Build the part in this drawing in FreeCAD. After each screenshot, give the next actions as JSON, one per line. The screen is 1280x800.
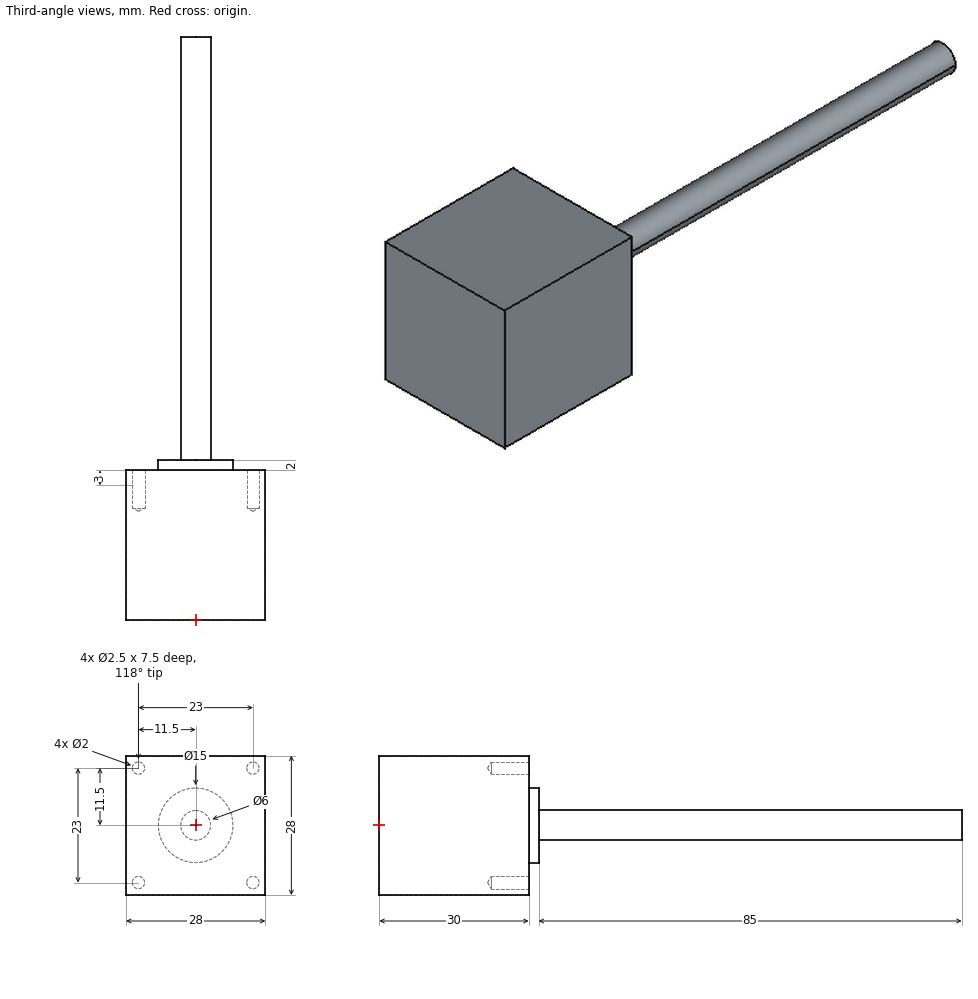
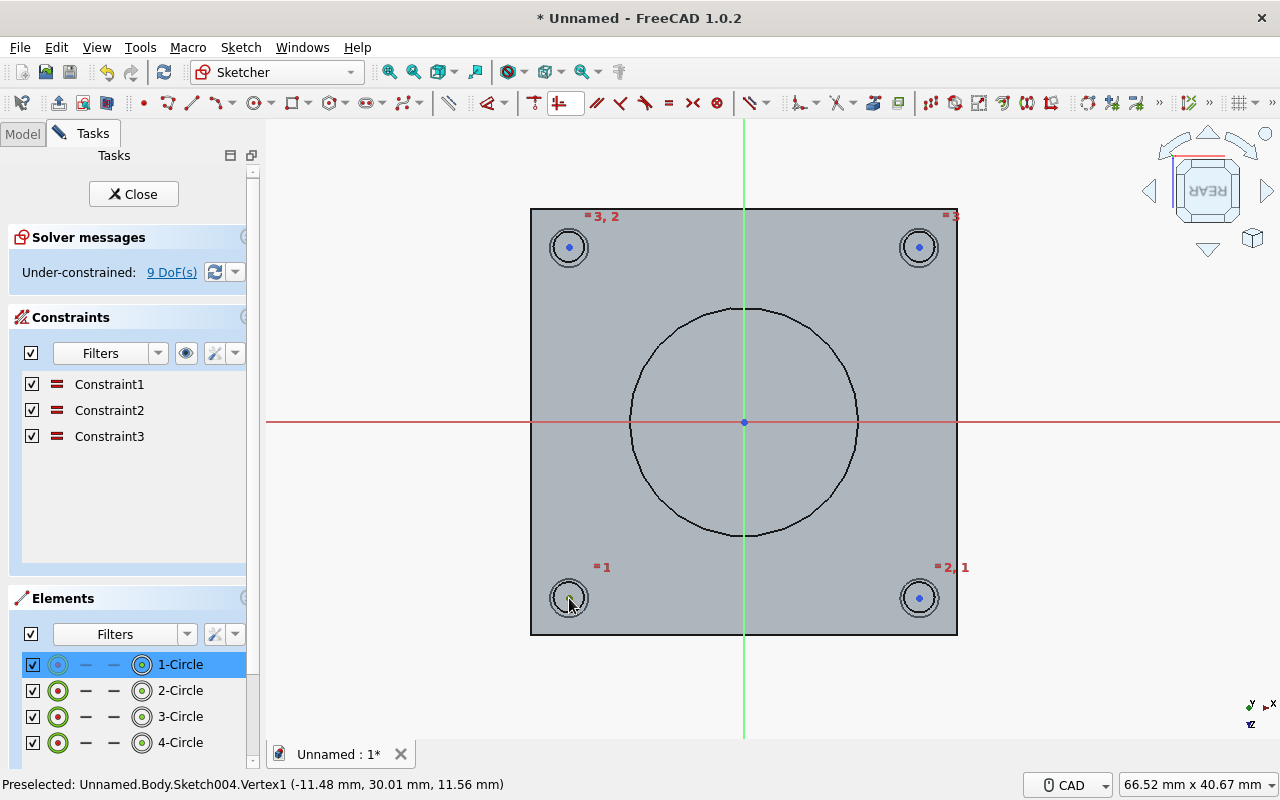
{"action": "left_click", "coordinate": [920, 598]}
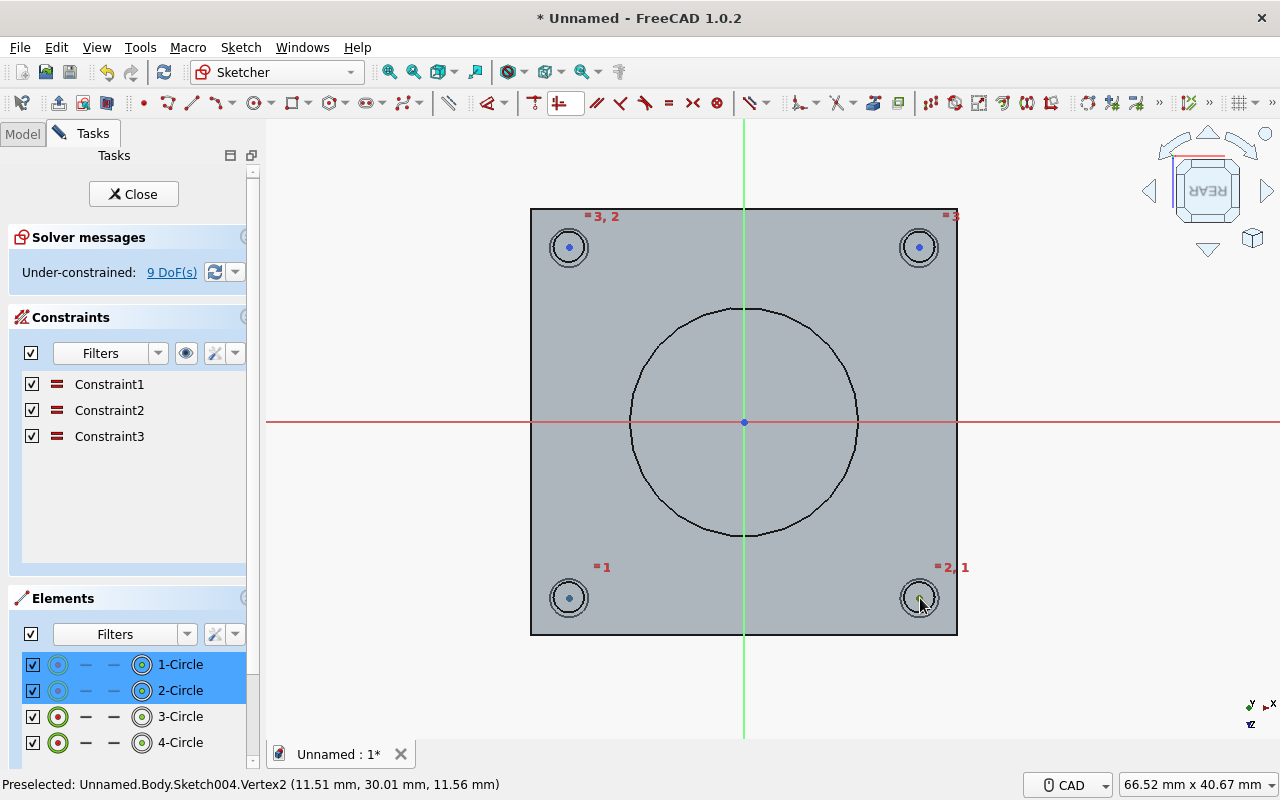
{"action": "left_click", "coordinate": [578, 104]}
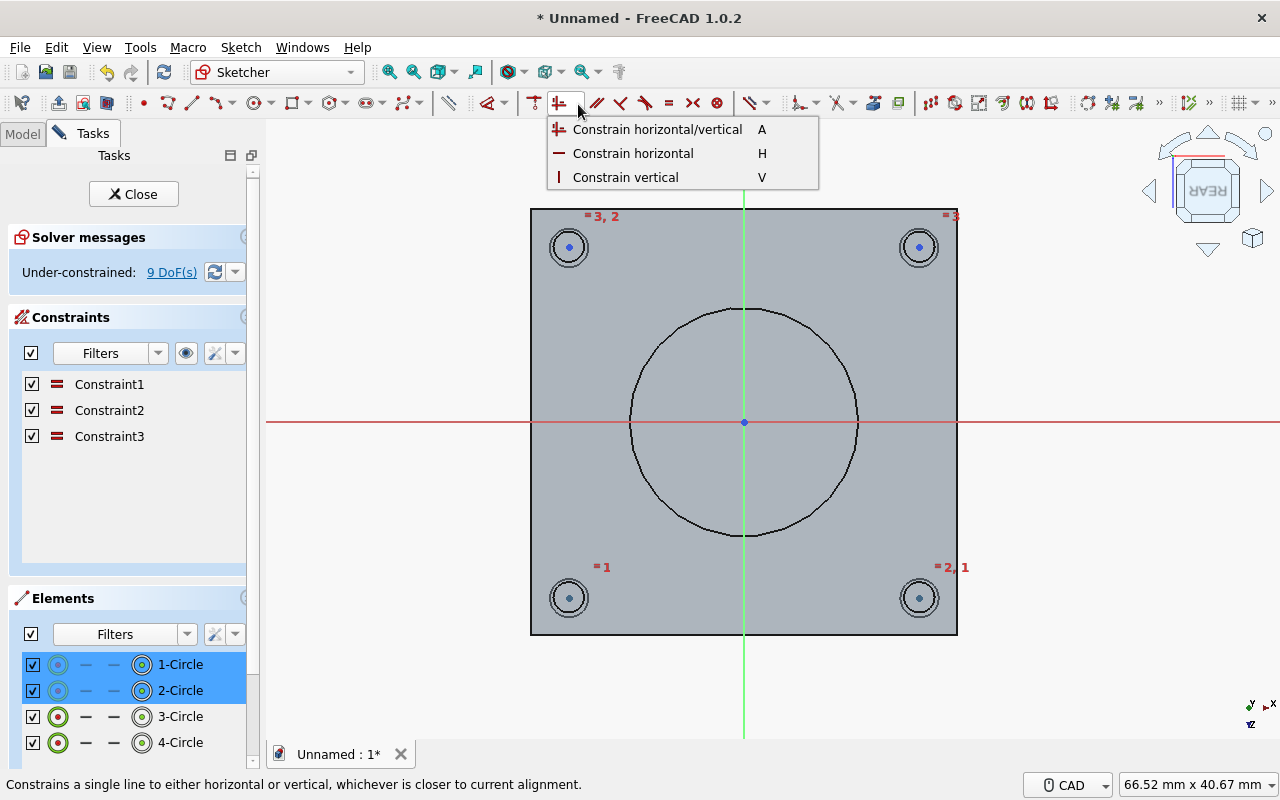
{"action": "left_click", "coordinate": [683, 153]}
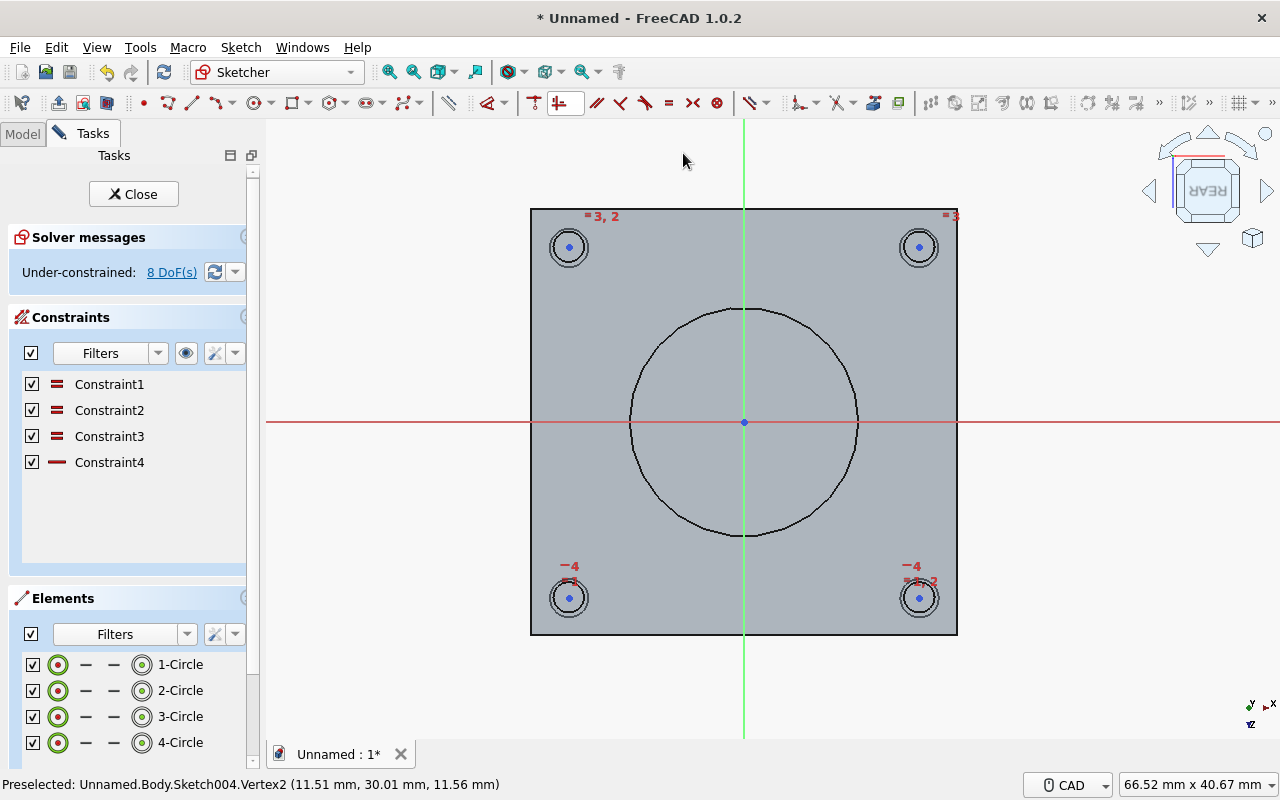
{"action": "left_click", "coordinate": [569, 598]}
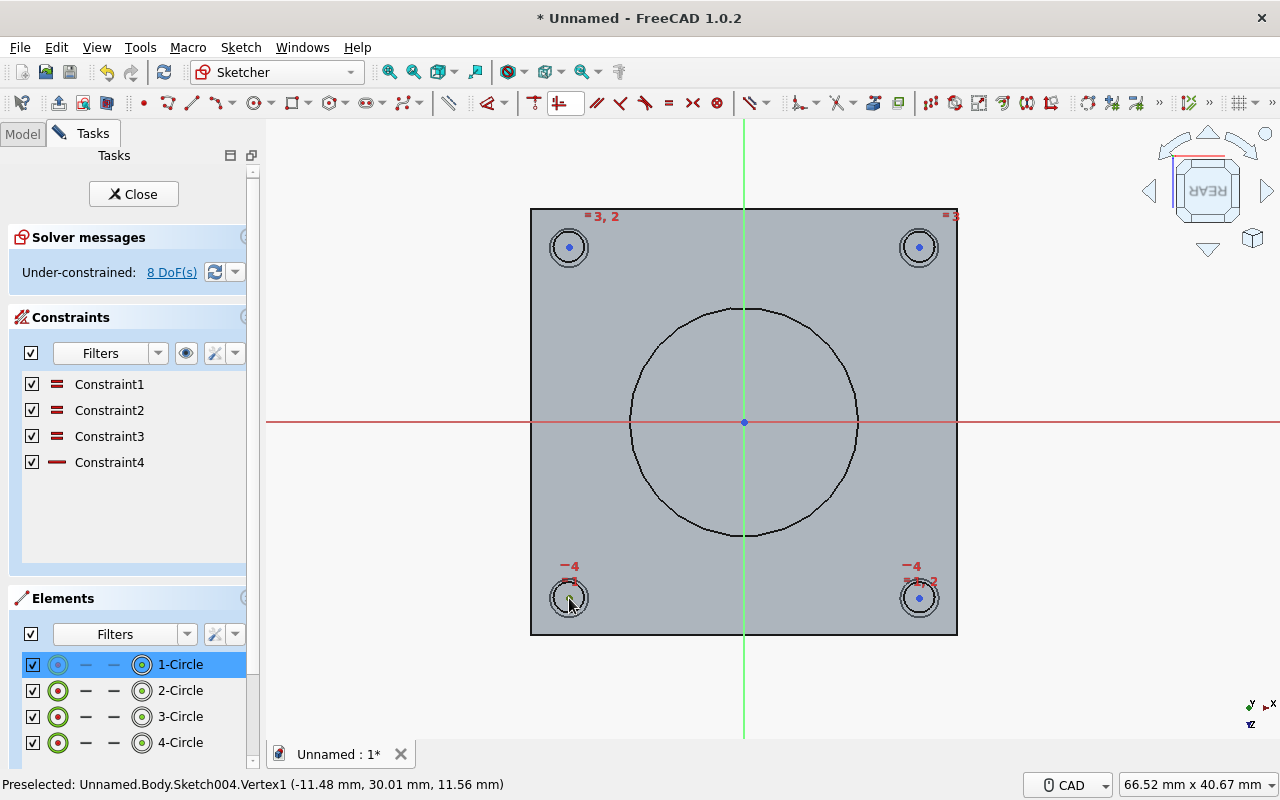
{"action": "left_click", "coordinate": [569, 248]}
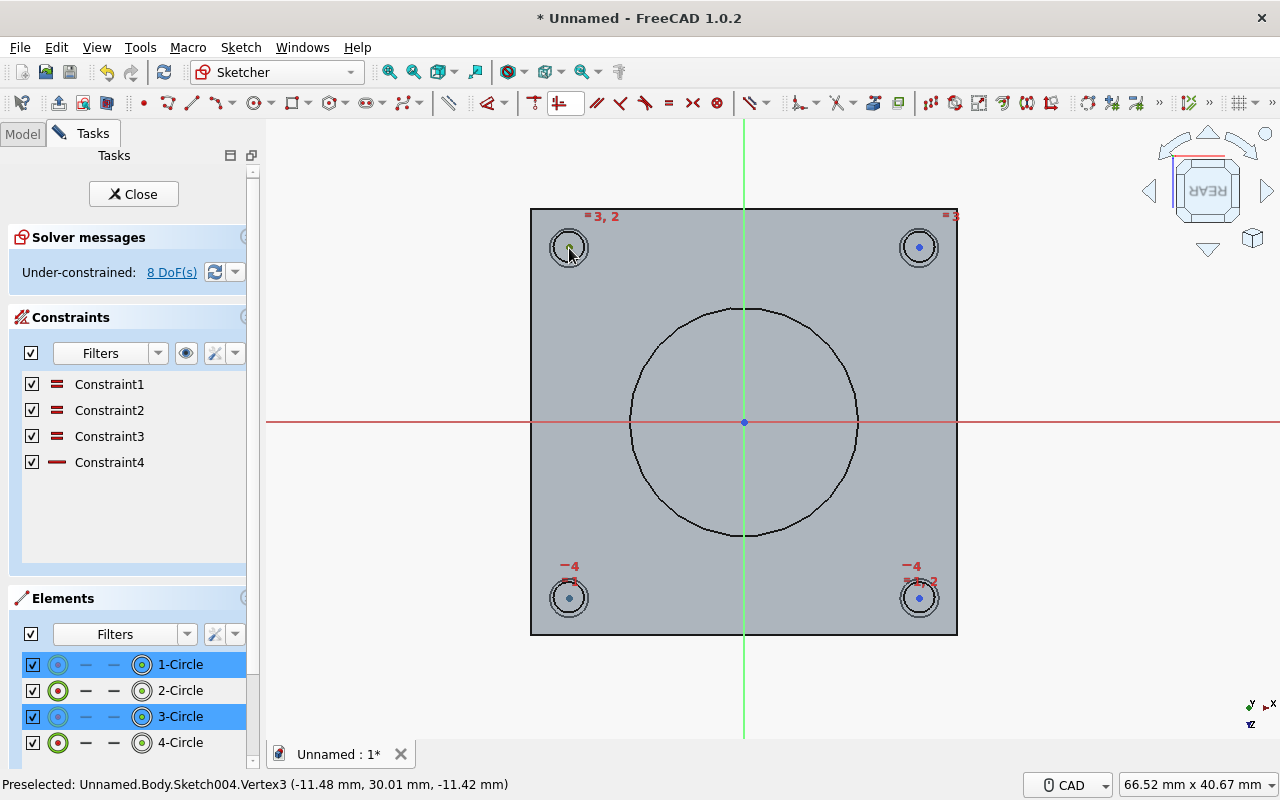
{"action": "key", "text": "v"}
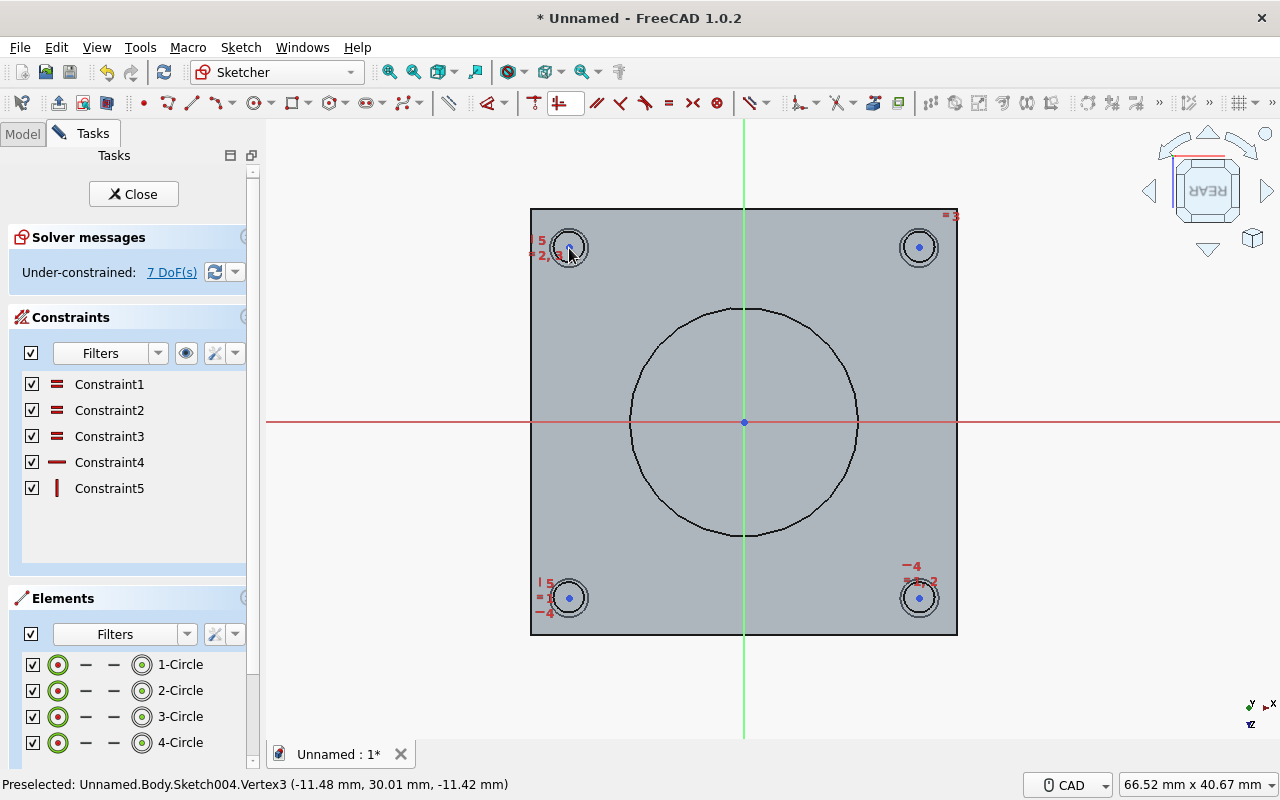
{"action": "left_click", "coordinate": [920, 598]}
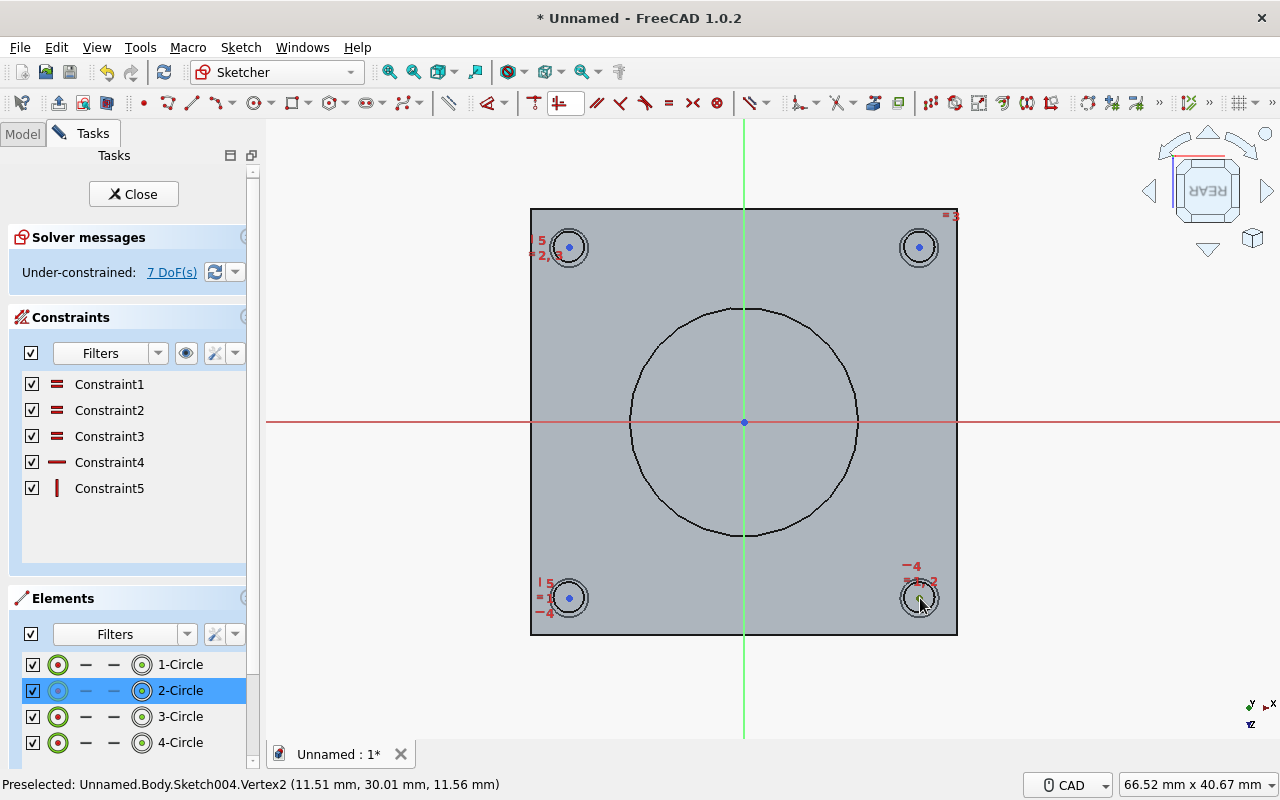
{"action": "left_click", "coordinate": [919, 248]}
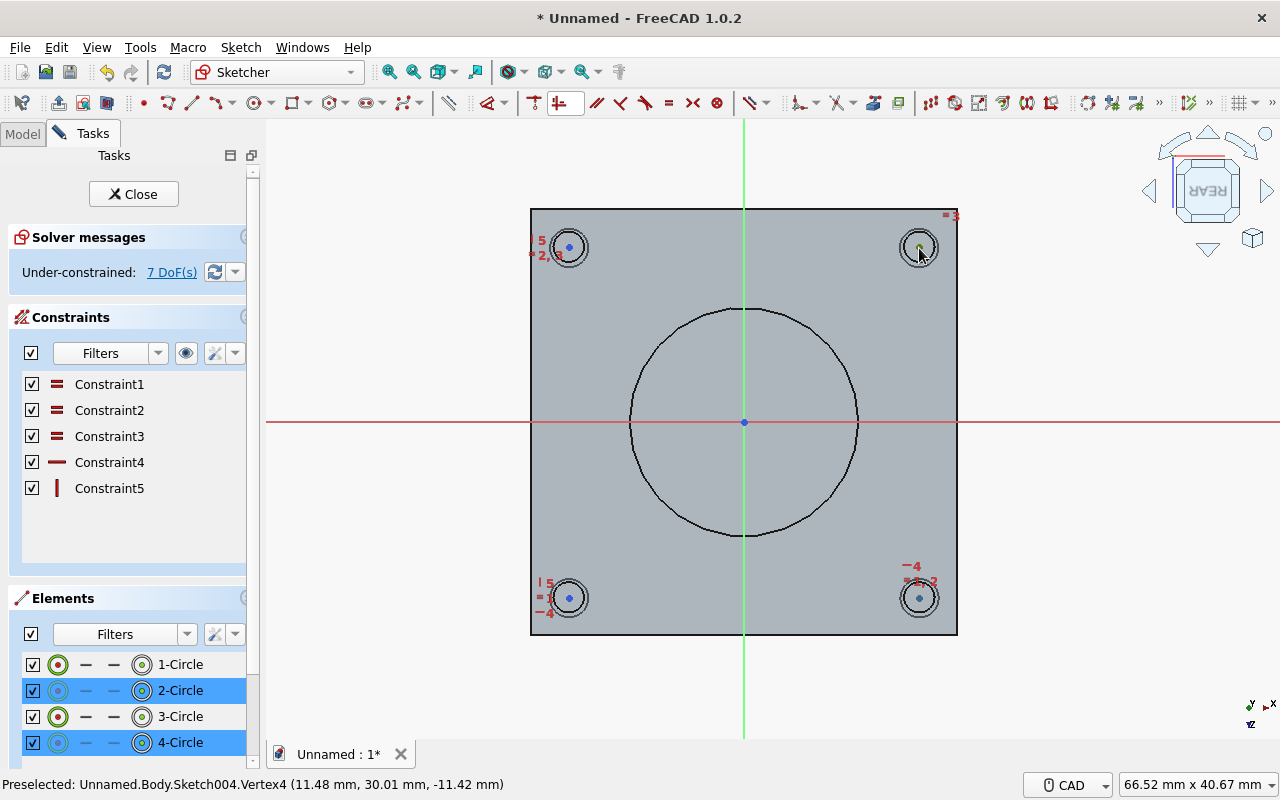
{"action": "left_click", "coordinate": [578, 104]}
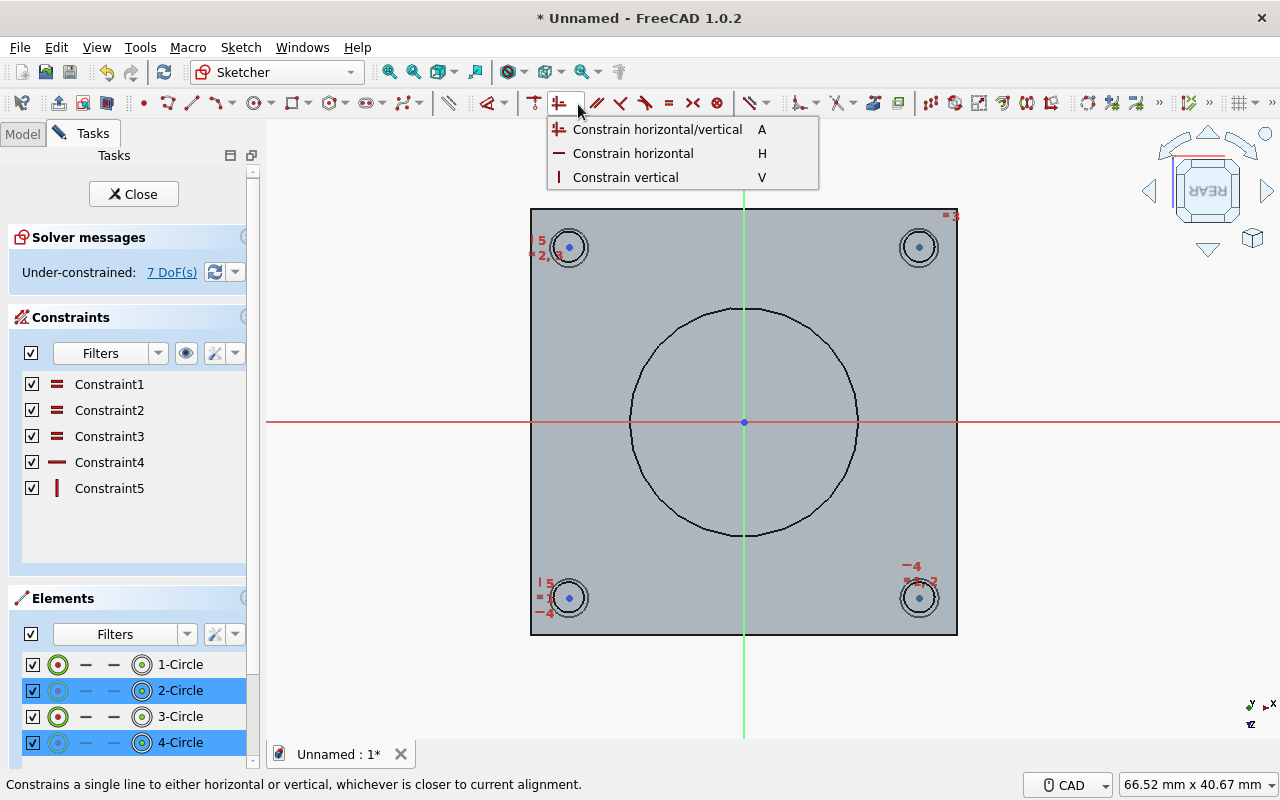
{"action": "left_click", "coordinate": [683, 177]}